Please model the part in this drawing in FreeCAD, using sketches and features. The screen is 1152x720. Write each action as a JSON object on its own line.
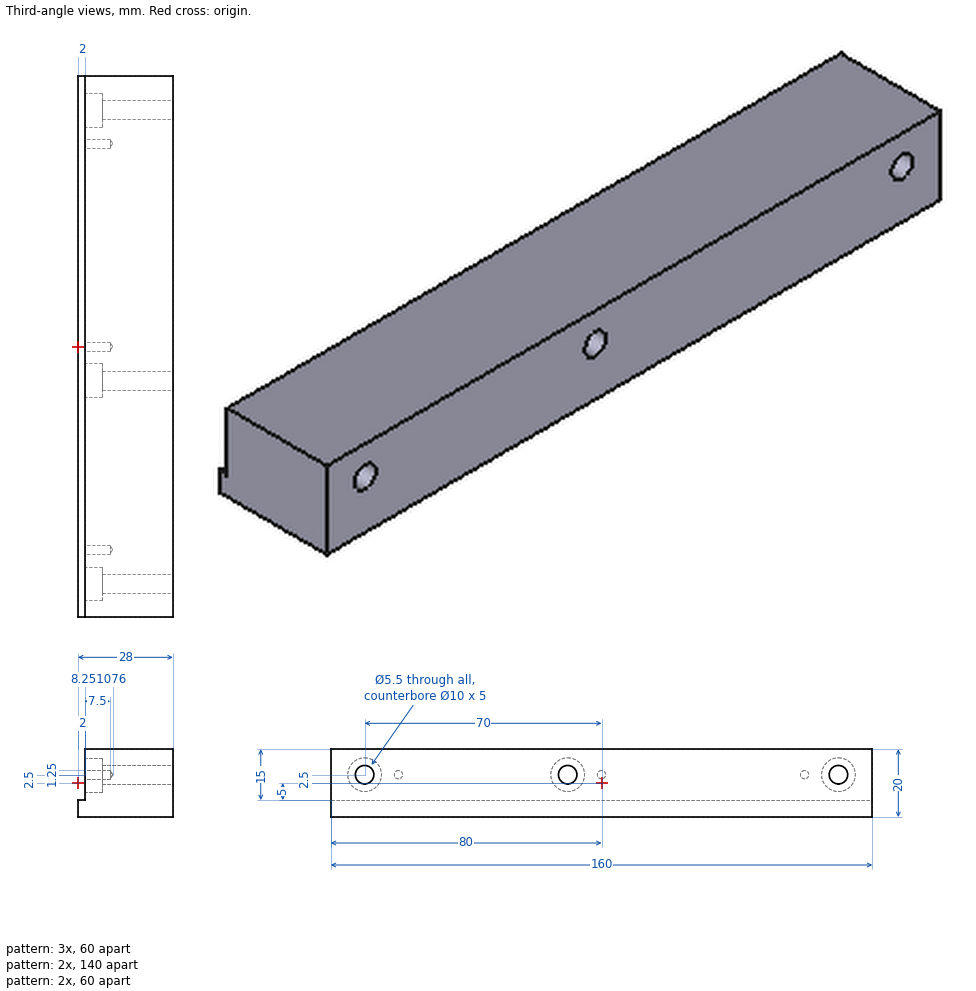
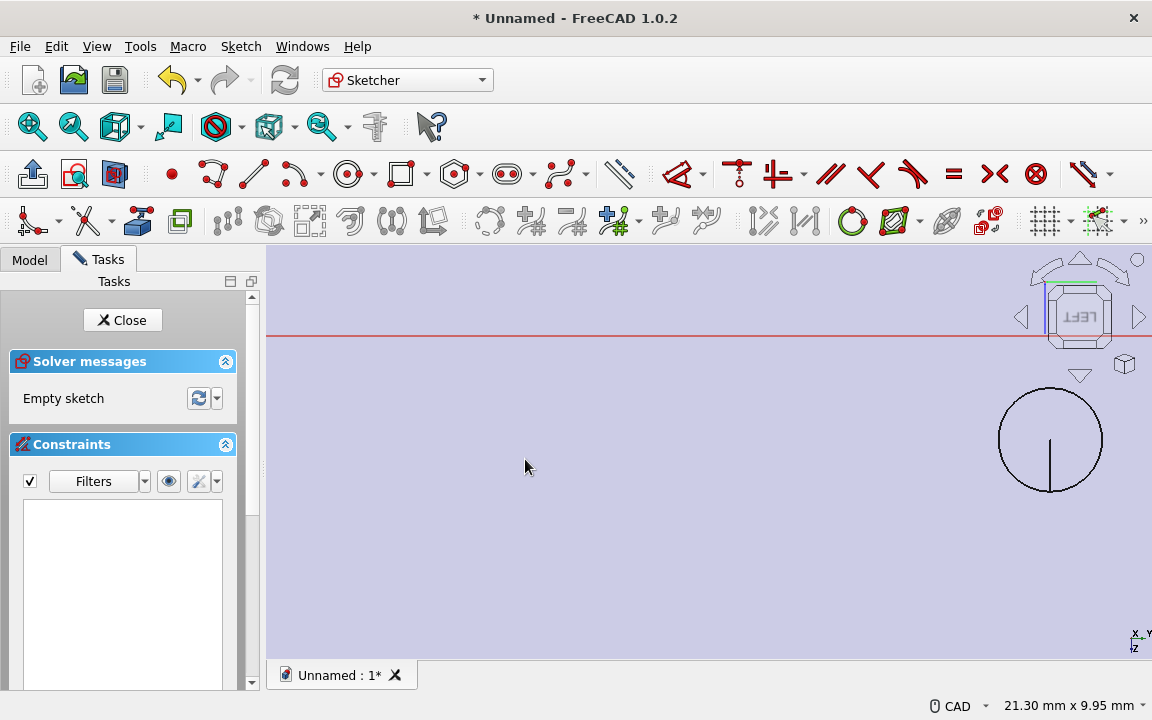
{"action": "key", "text": "g c"}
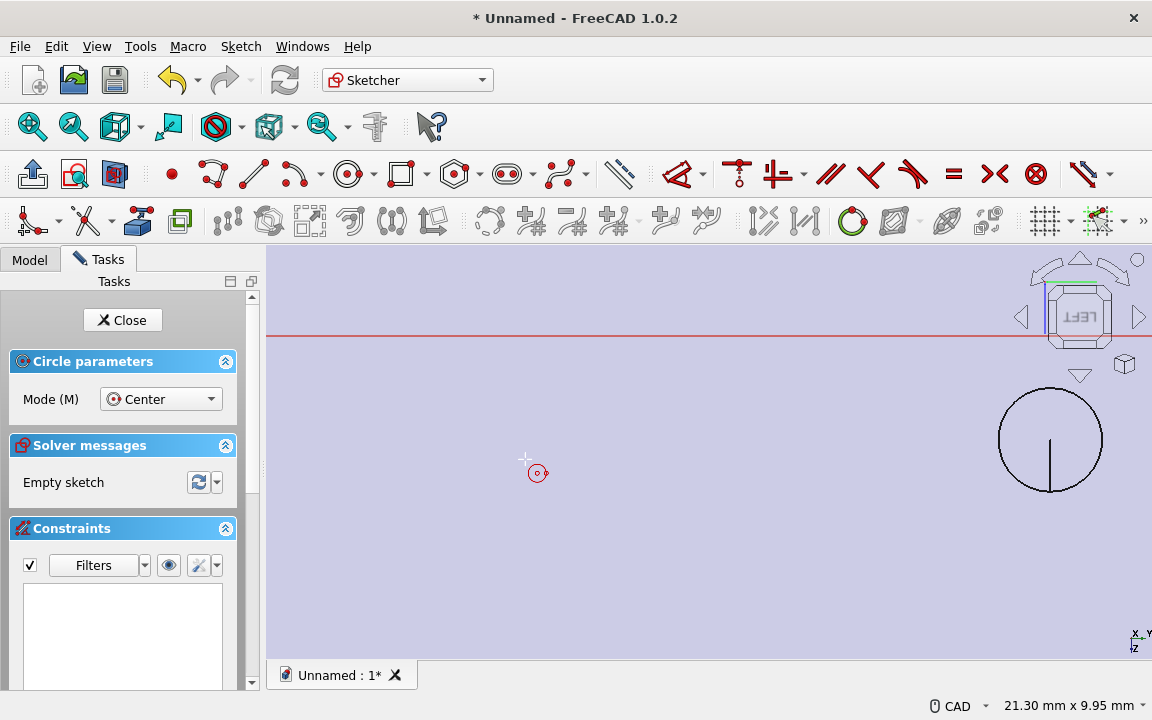
{"action": "left_click", "coordinate": [634, 440]}
{"action": "left_click", "coordinate": [715, 359]}
{"action": "key", "text": "Escape"}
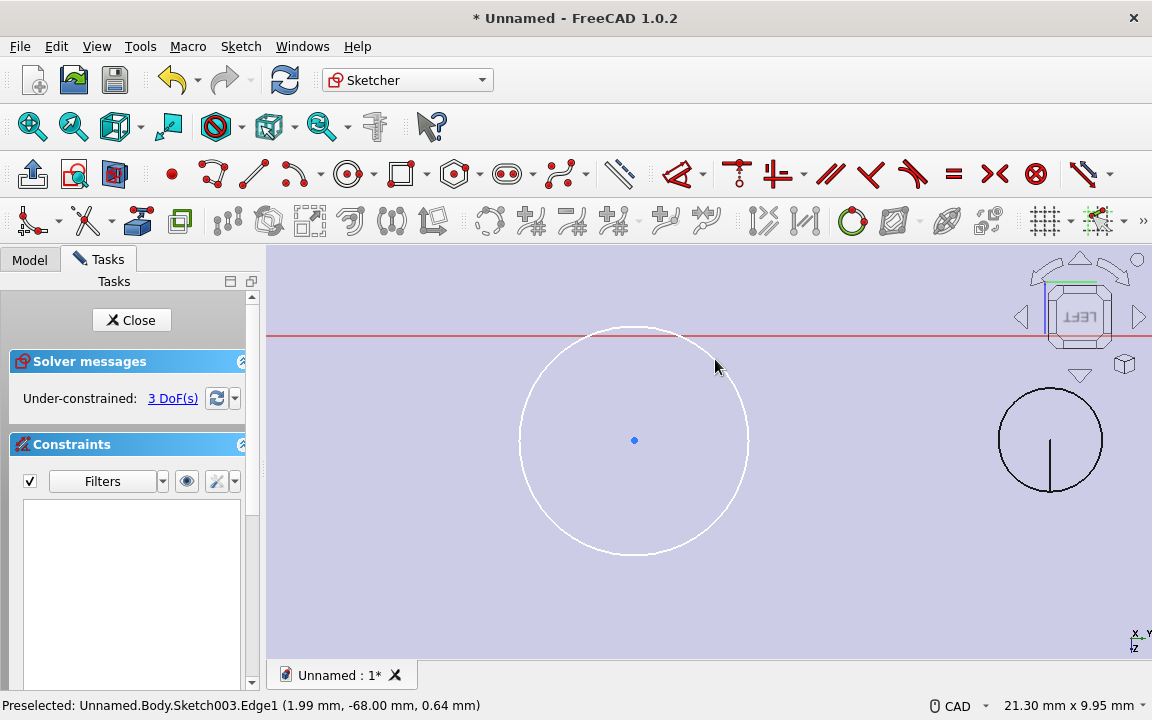
{"action": "key", "text": "d"}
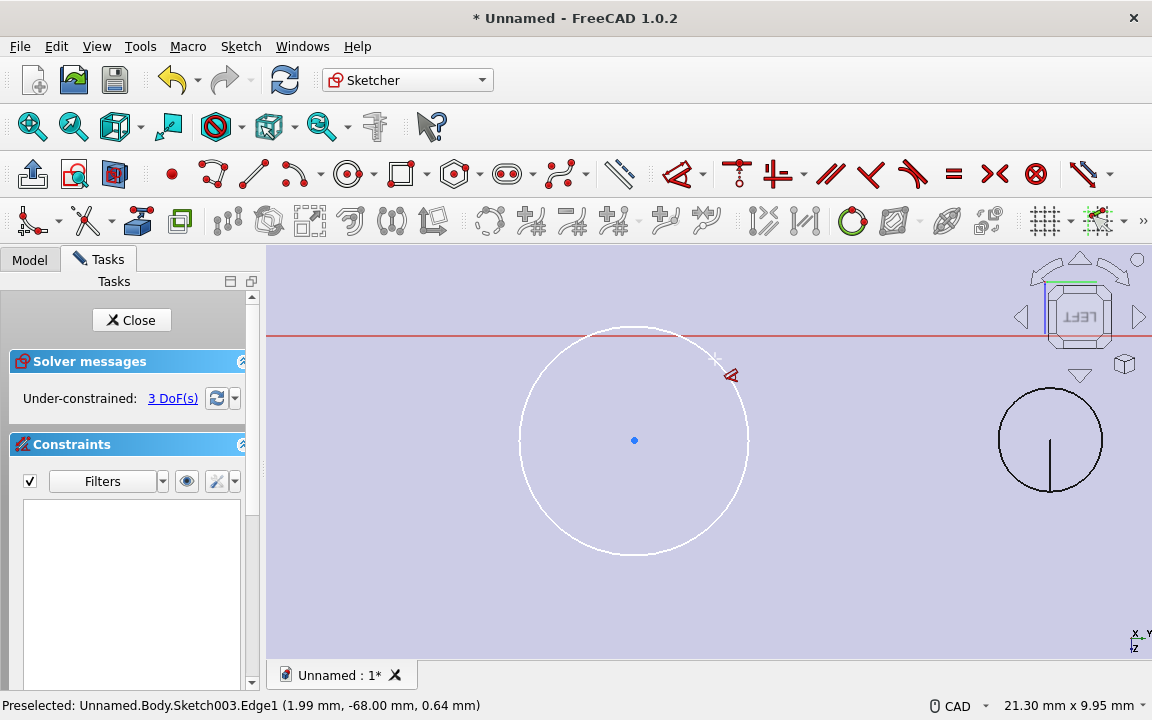
{"action": "left_click", "coordinate": [715, 360]}
{"action": "left_click", "coordinate": [775, 400]}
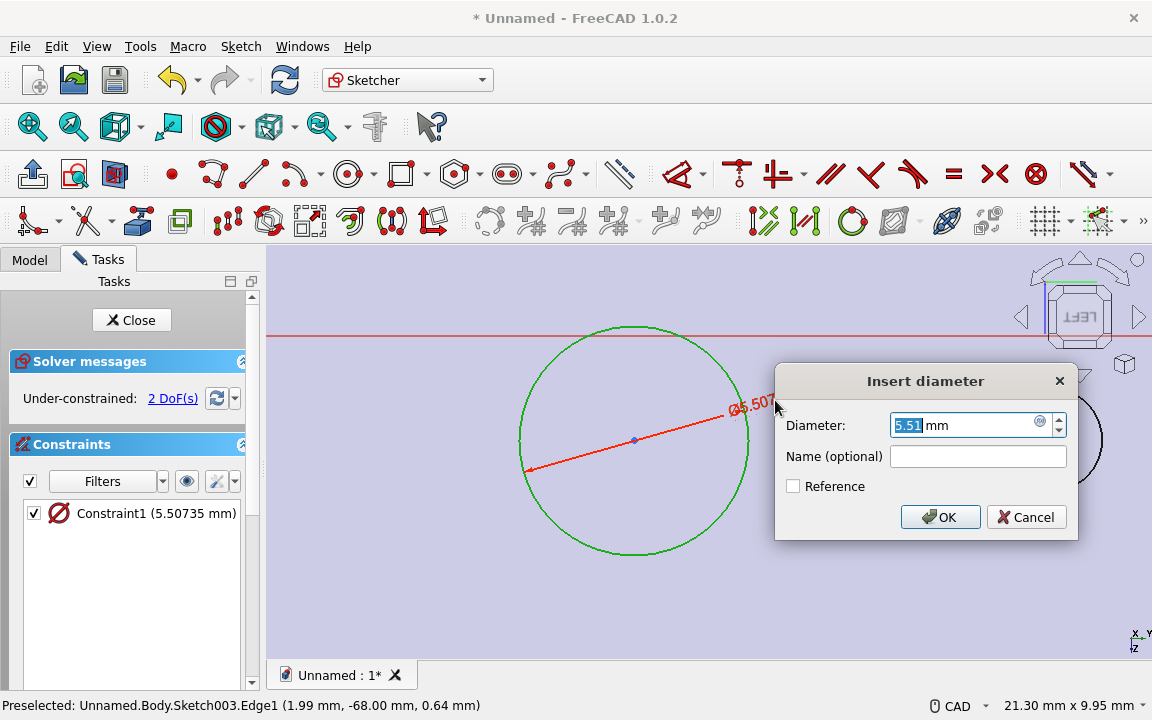
{"action": "type", "text": "5.5"}
{"action": "key", "text": "Return"}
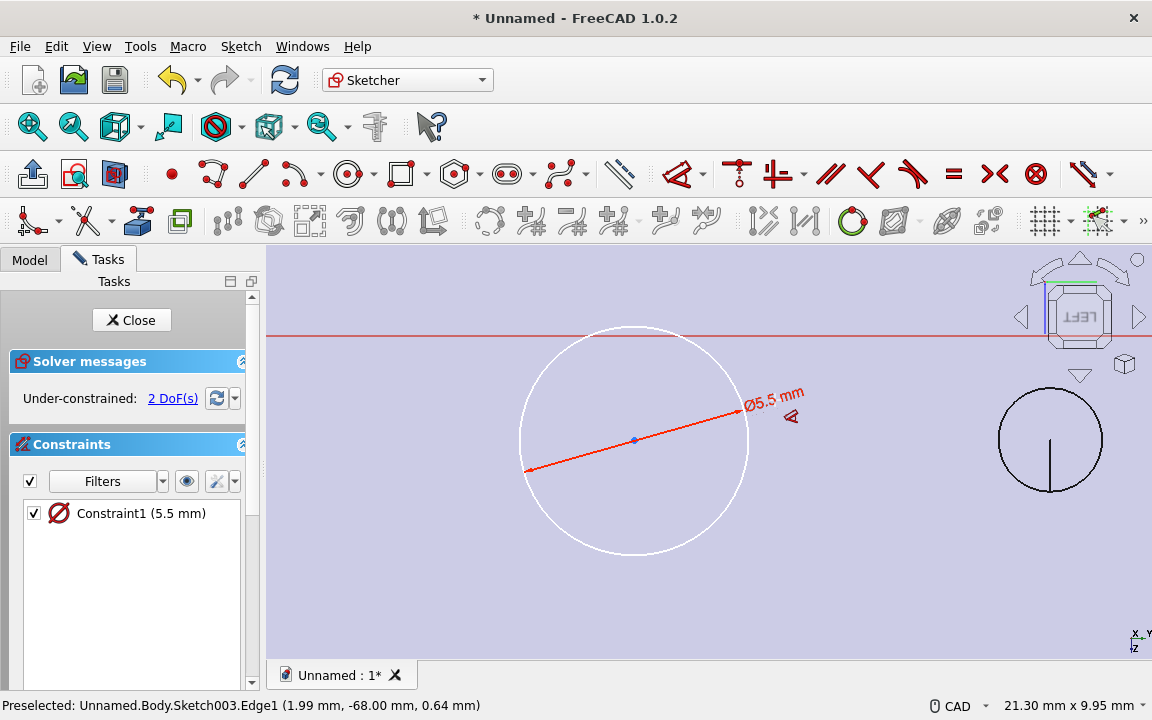
{"action": "left_click", "coordinate": [634, 441]}
{"action": "left_click", "coordinate": [811, 302]}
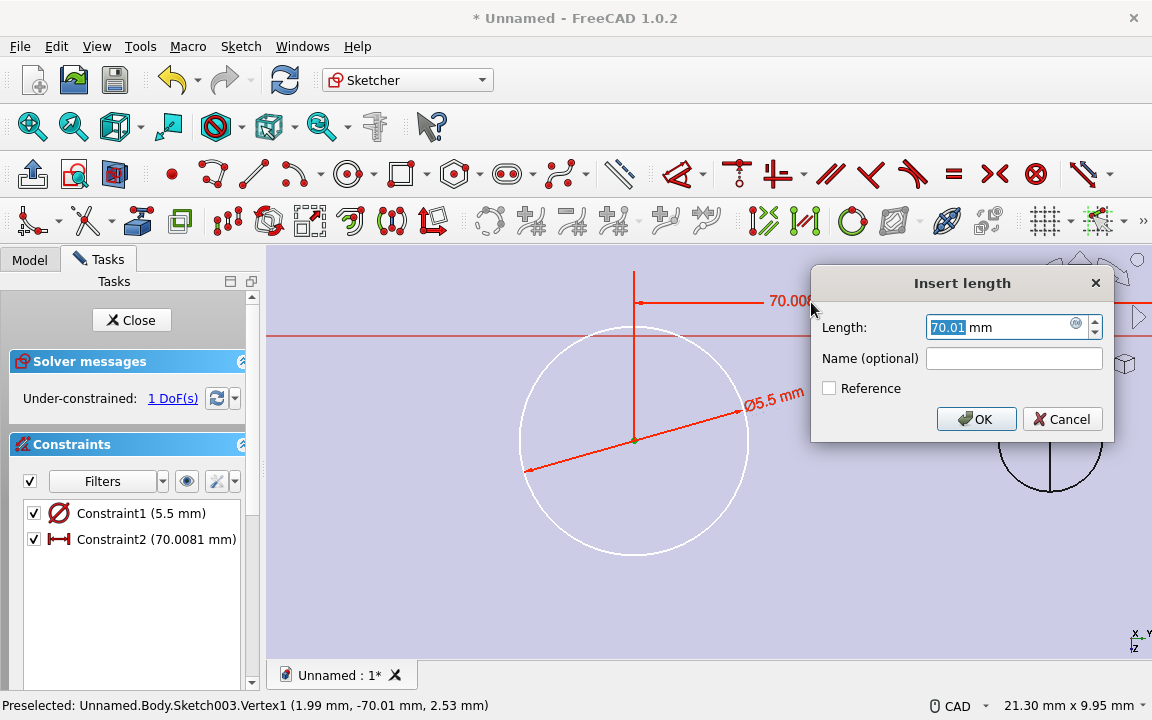
{"action": "type", "text": "70"}
{"action": "key", "text": "Return"}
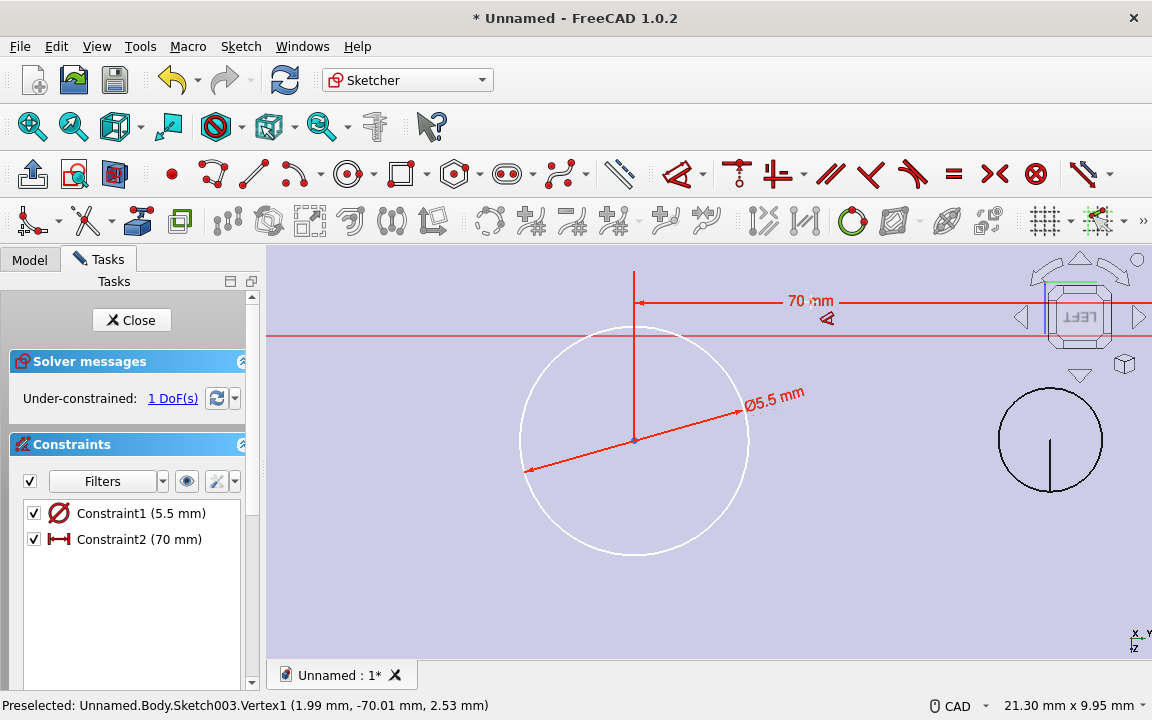
{"action": "left_click", "coordinate": [634, 441]}
{"action": "left_click", "coordinate": [600, 388]}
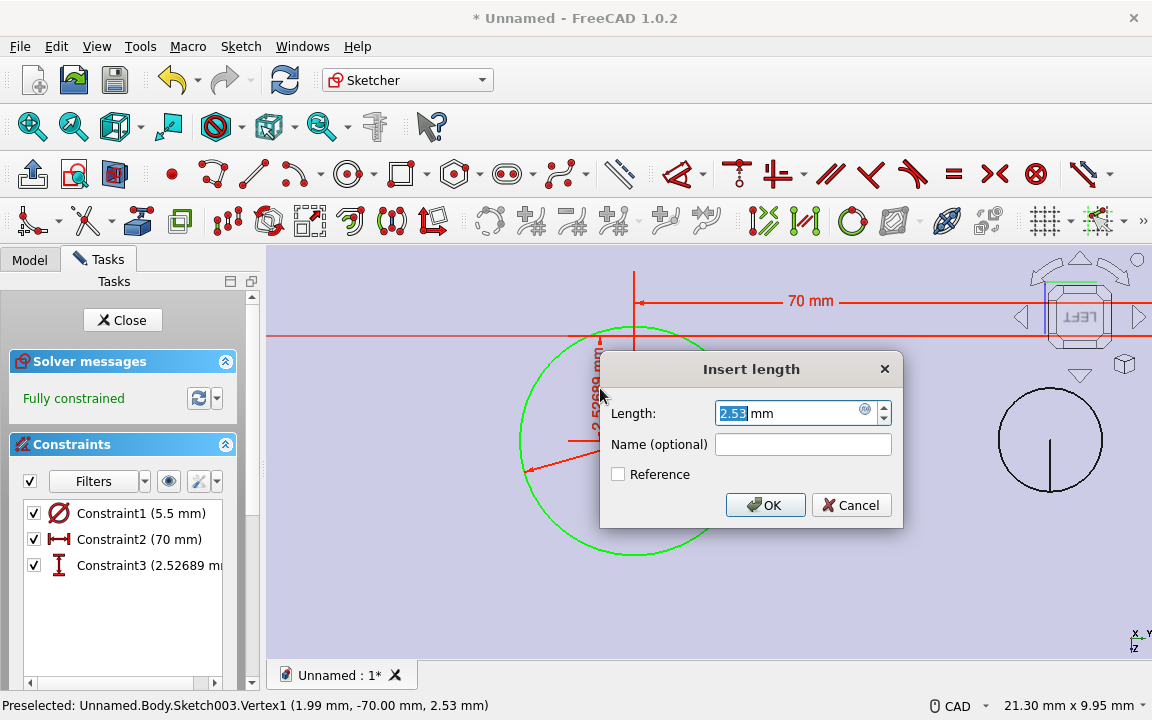
{"action": "type", "text": "2.5"}
{"action": "key", "text": "Return"}
{"action": "key", "text": "Escape"}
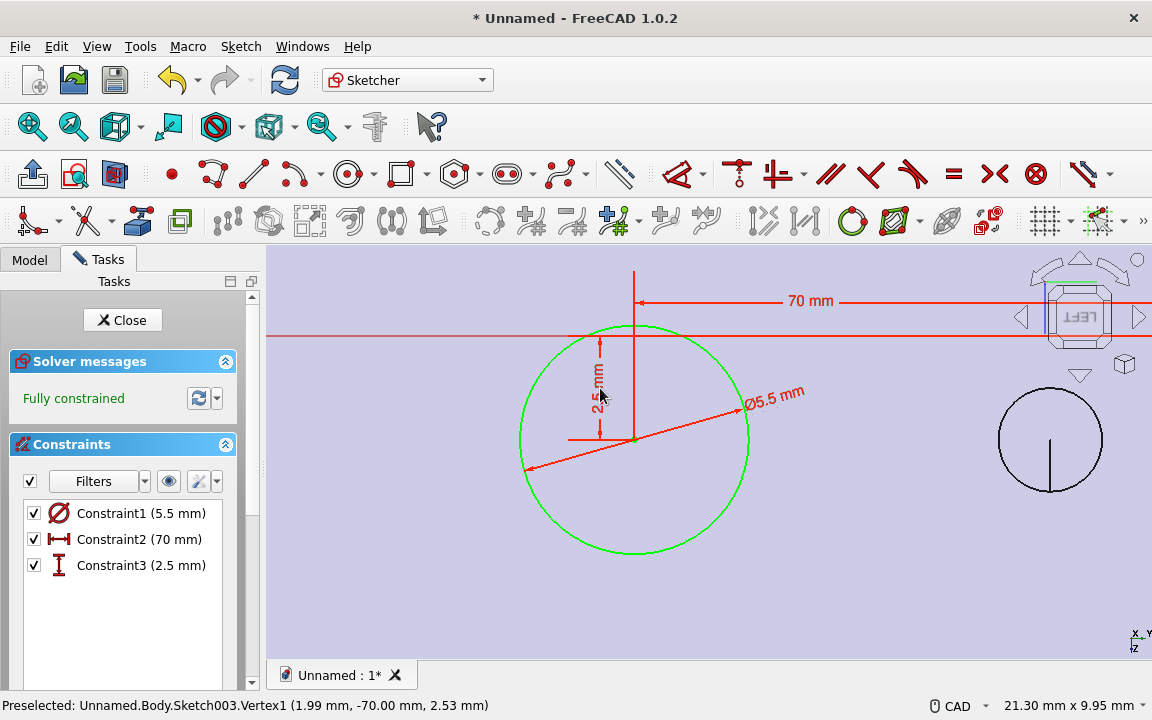
{"action": "left_click", "coordinate": [123, 320]}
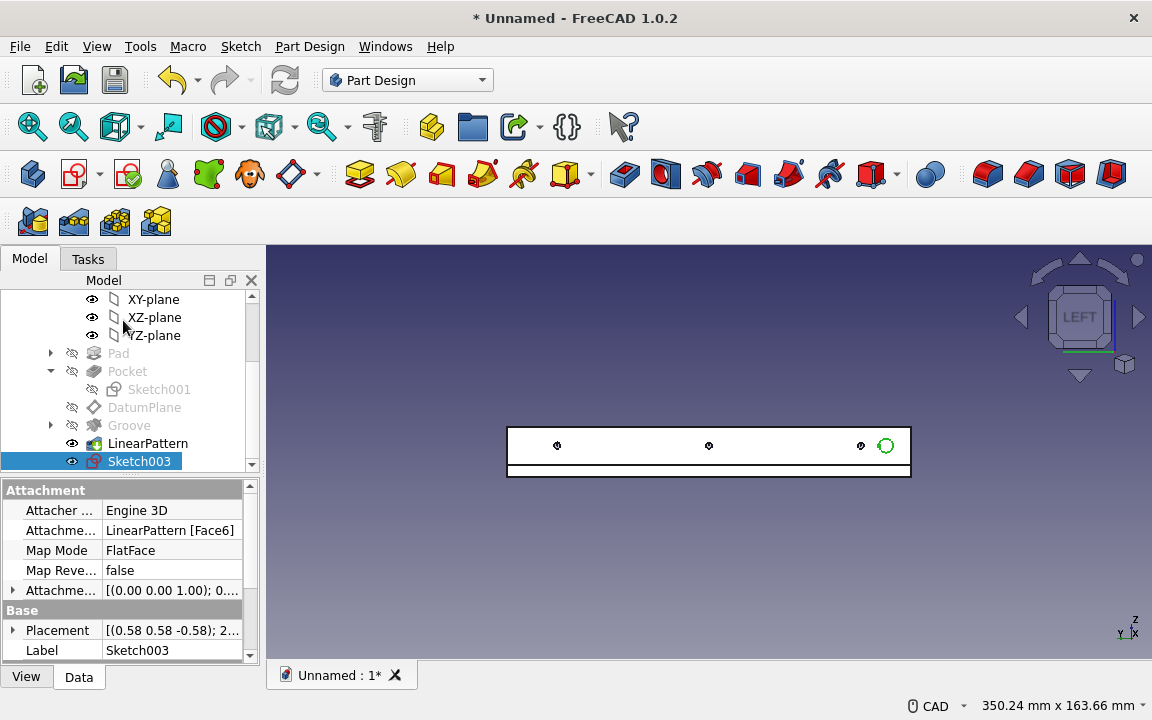
{"action": "left_click", "coordinate": [666, 174]}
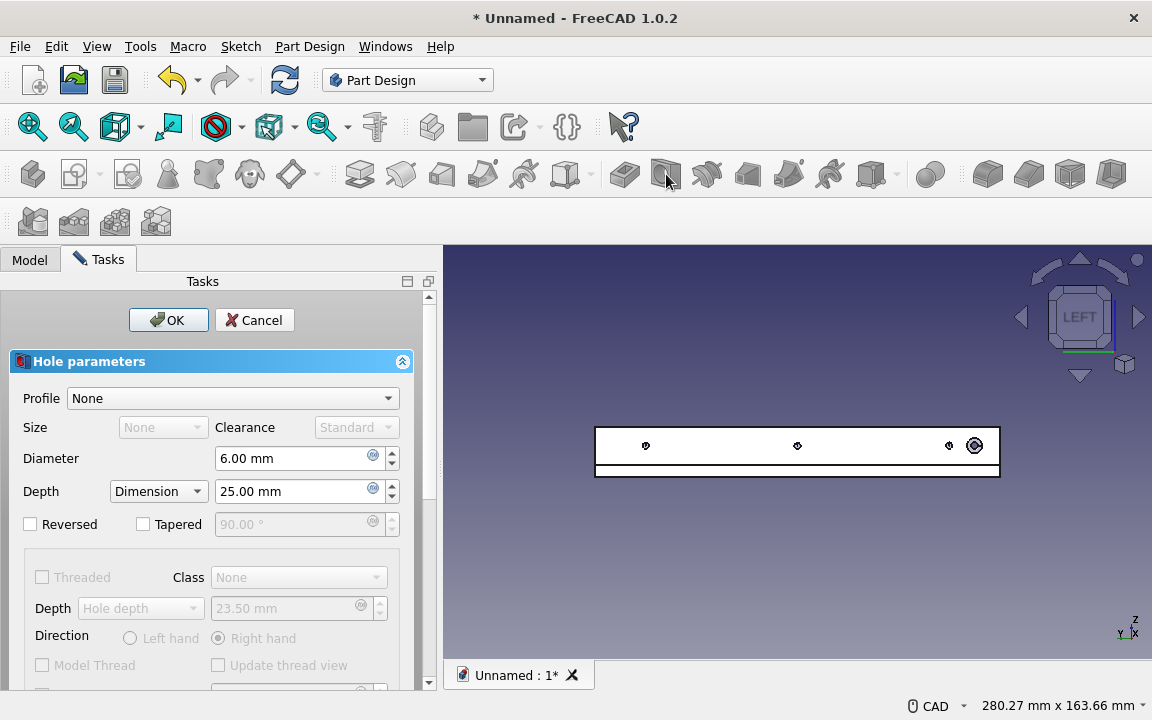
{"action": "triple_click", "coordinate": [300, 458]}